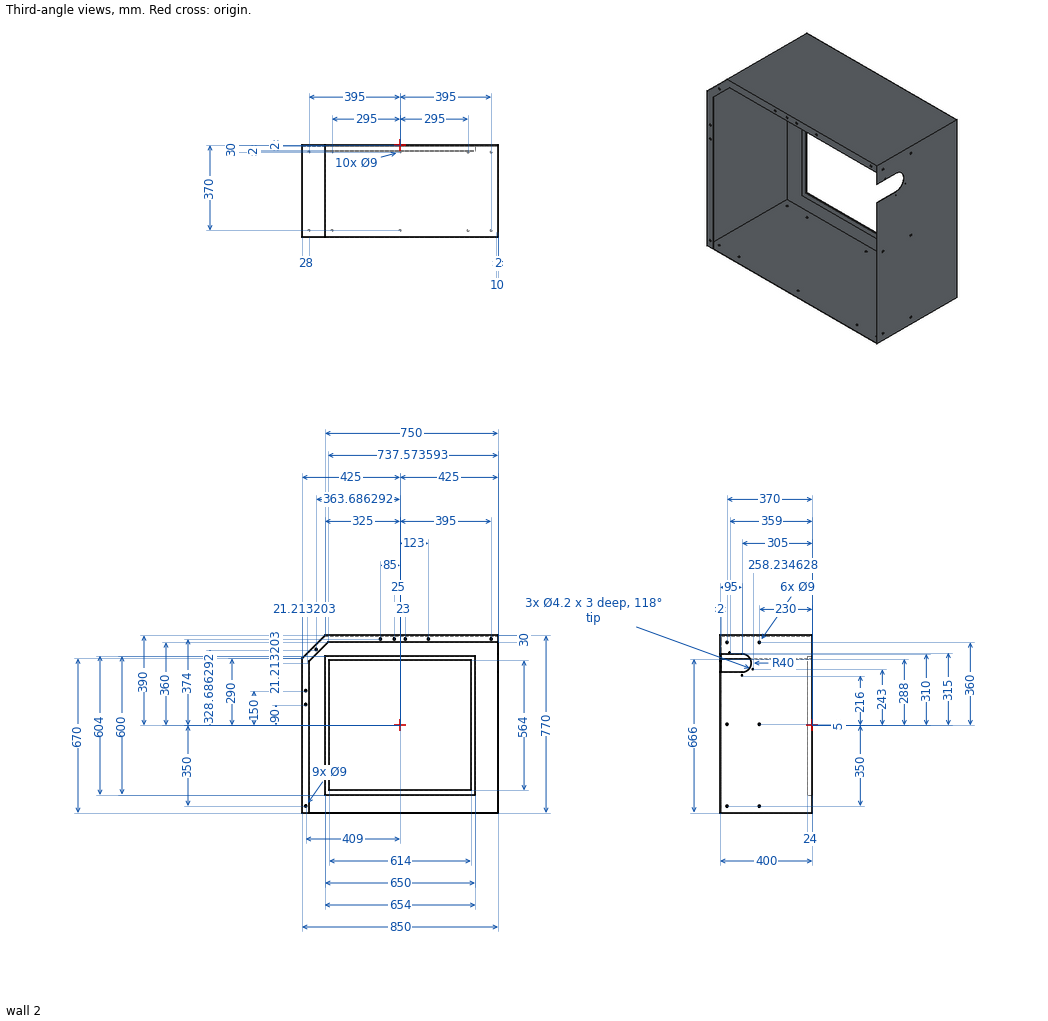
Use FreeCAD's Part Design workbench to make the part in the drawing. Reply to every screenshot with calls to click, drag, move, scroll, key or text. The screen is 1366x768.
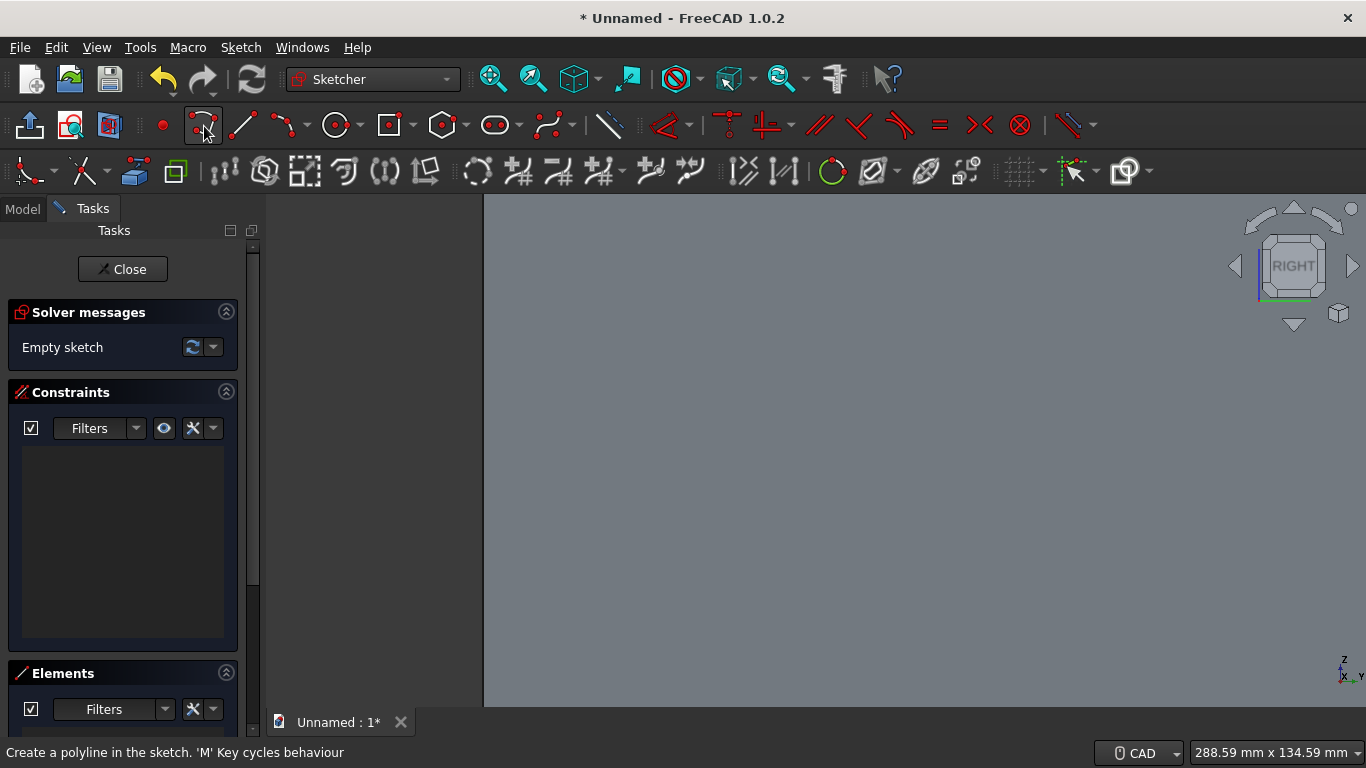
click(846, 293)
click(483, 293)
click(483, 598)
click(846, 598)
right_click(846, 598)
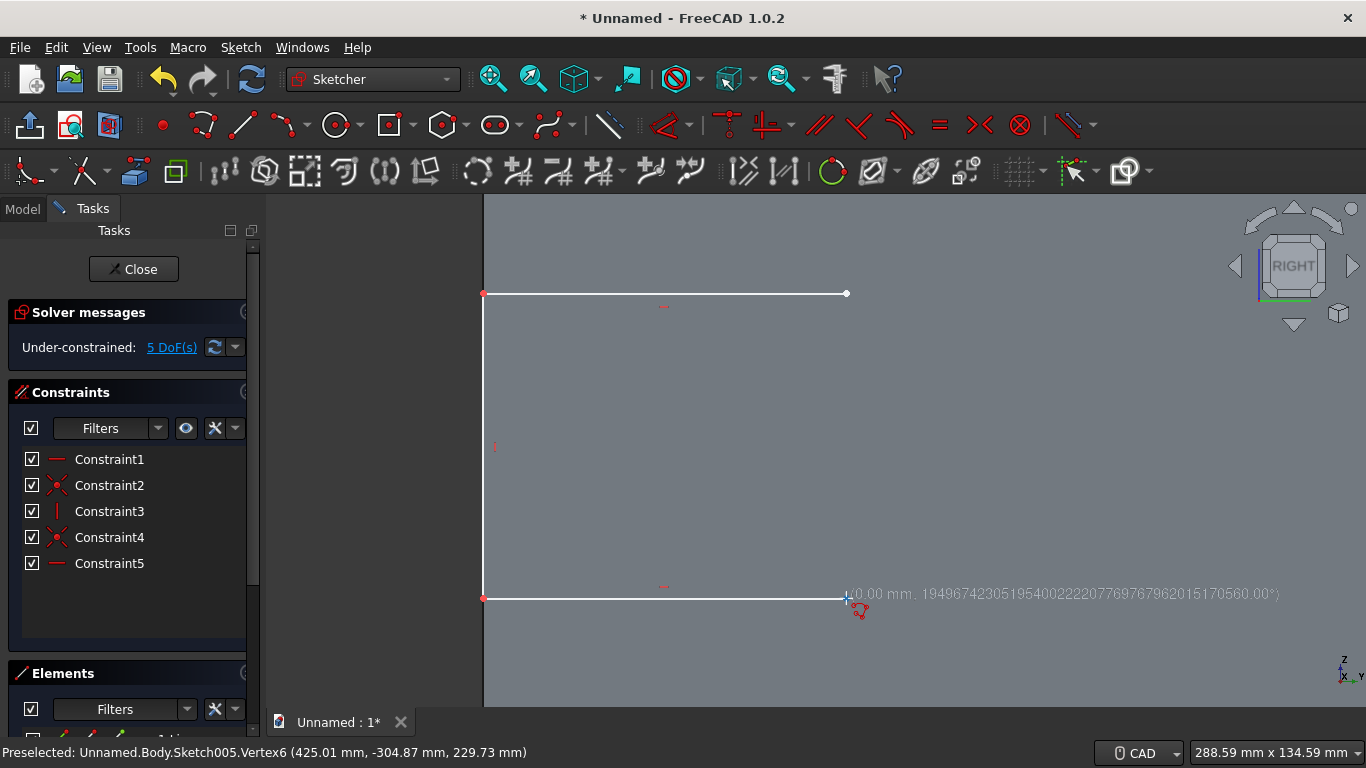
click(284, 126)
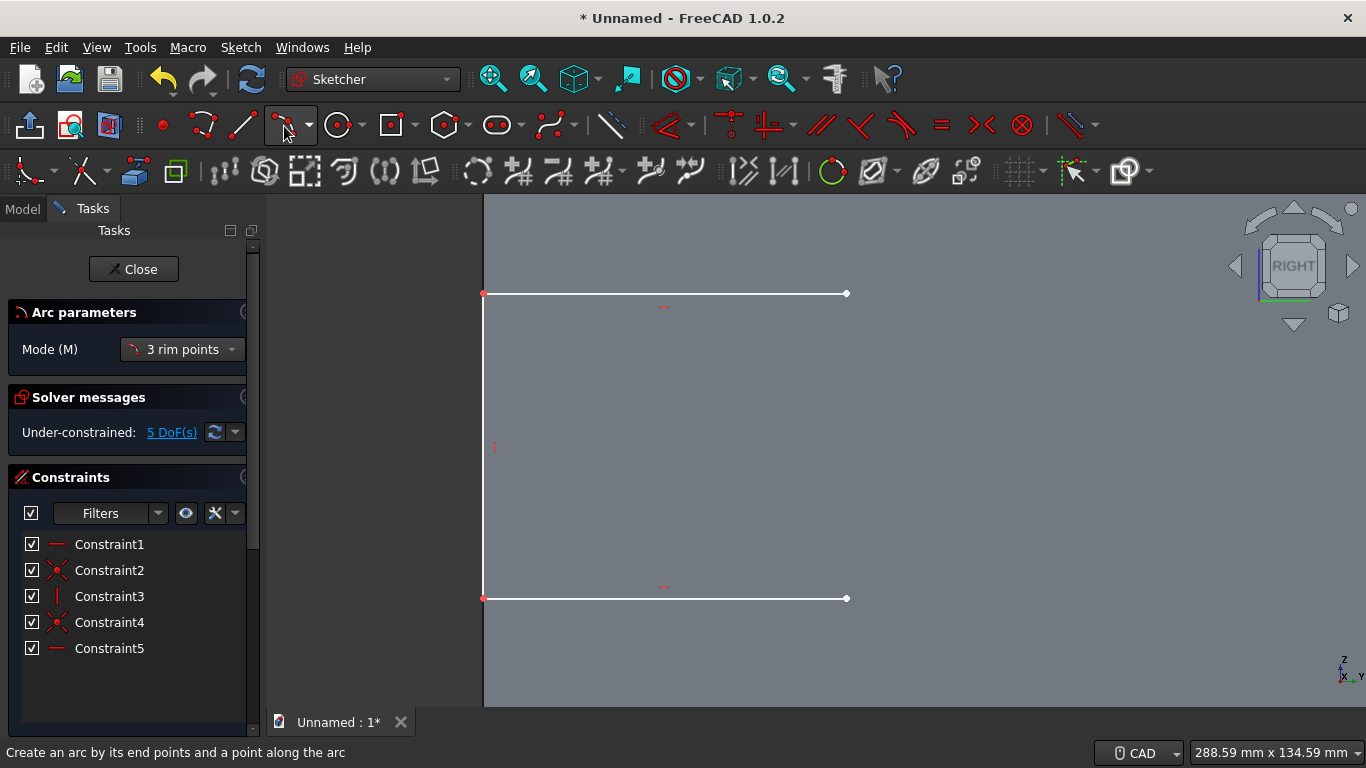
click(846, 599)
click(846, 294)
click(998, 446)
key(Escape)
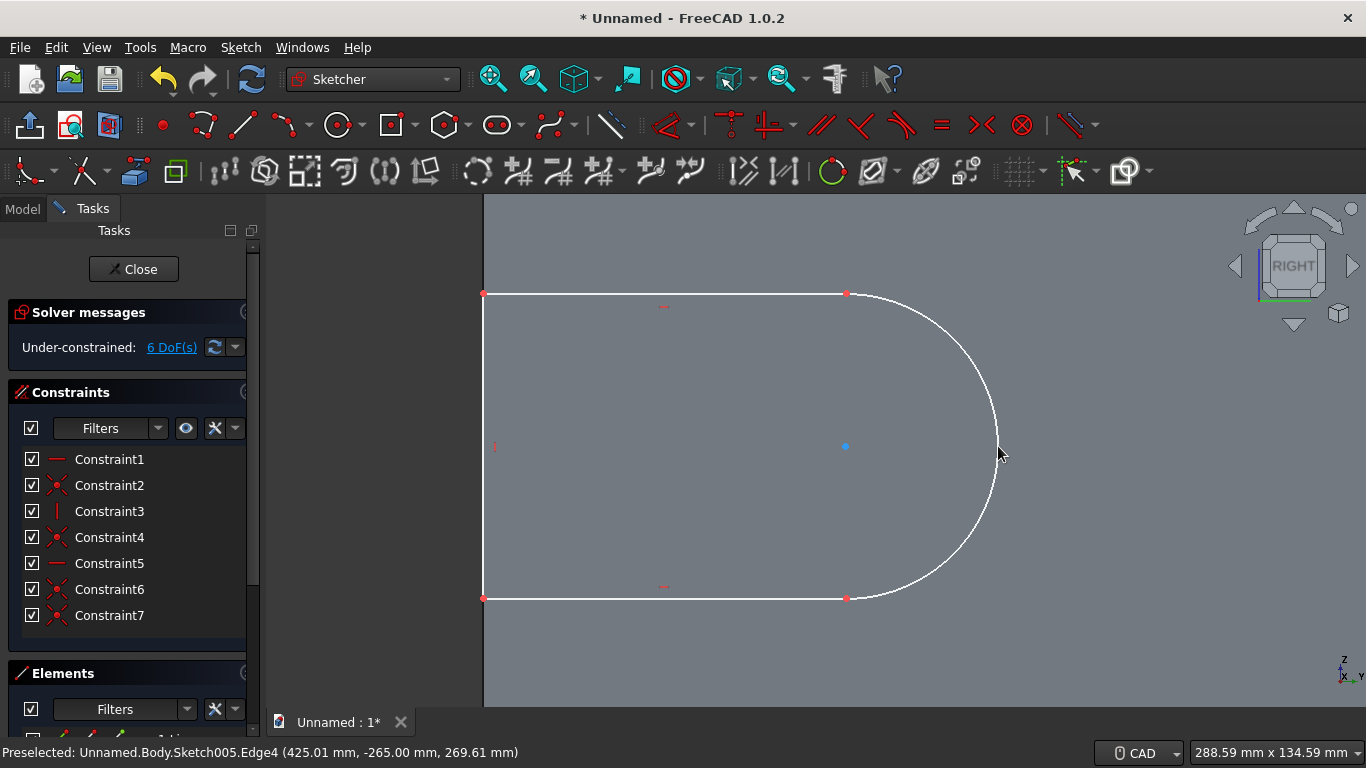
click(666, 126)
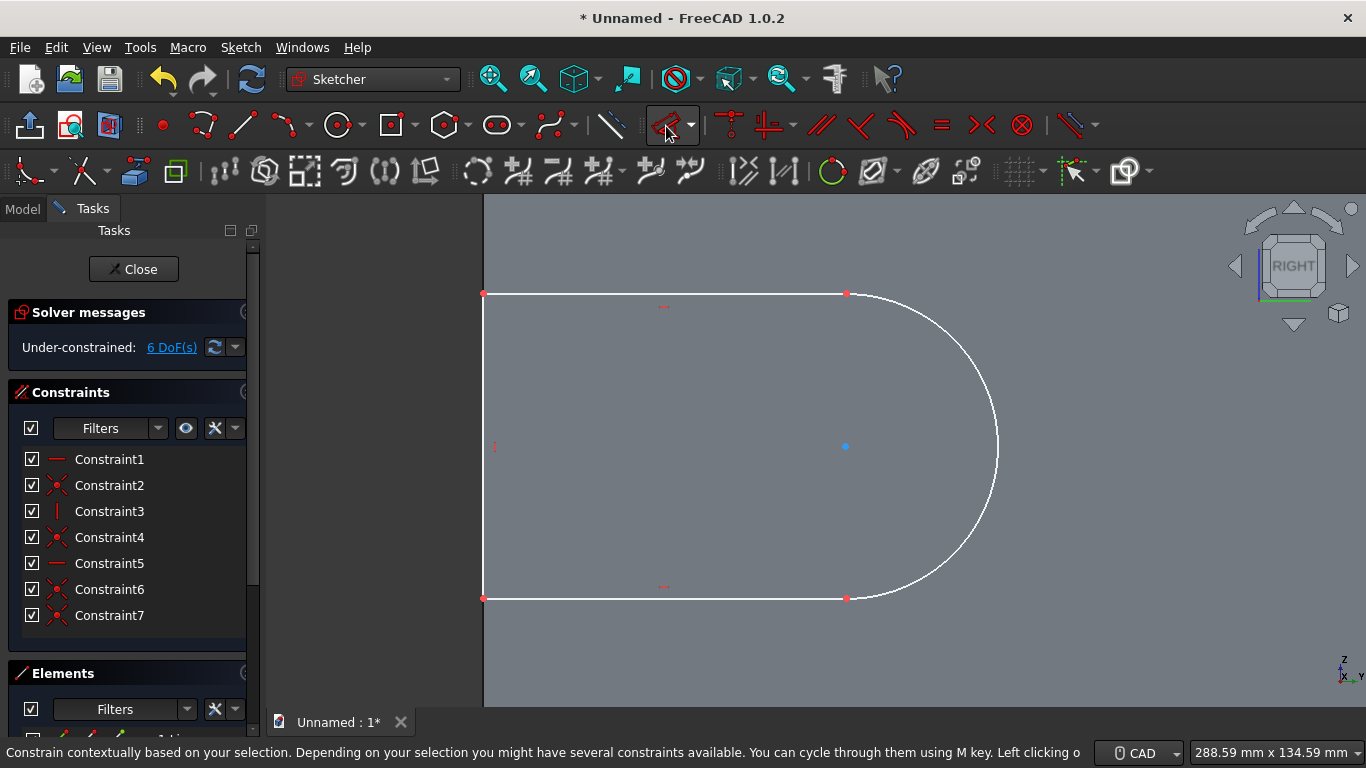
click(969, 536)
click(995, 555)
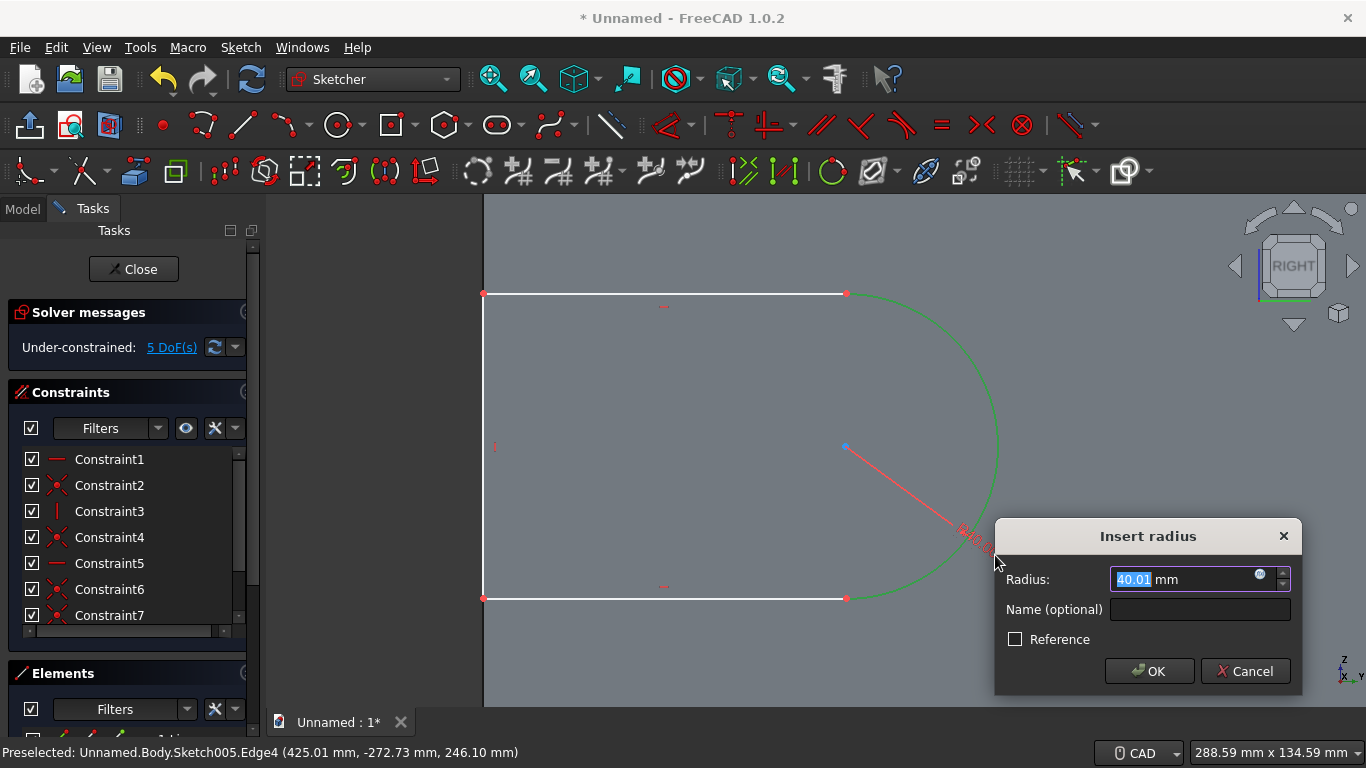
text(40)
key(Return)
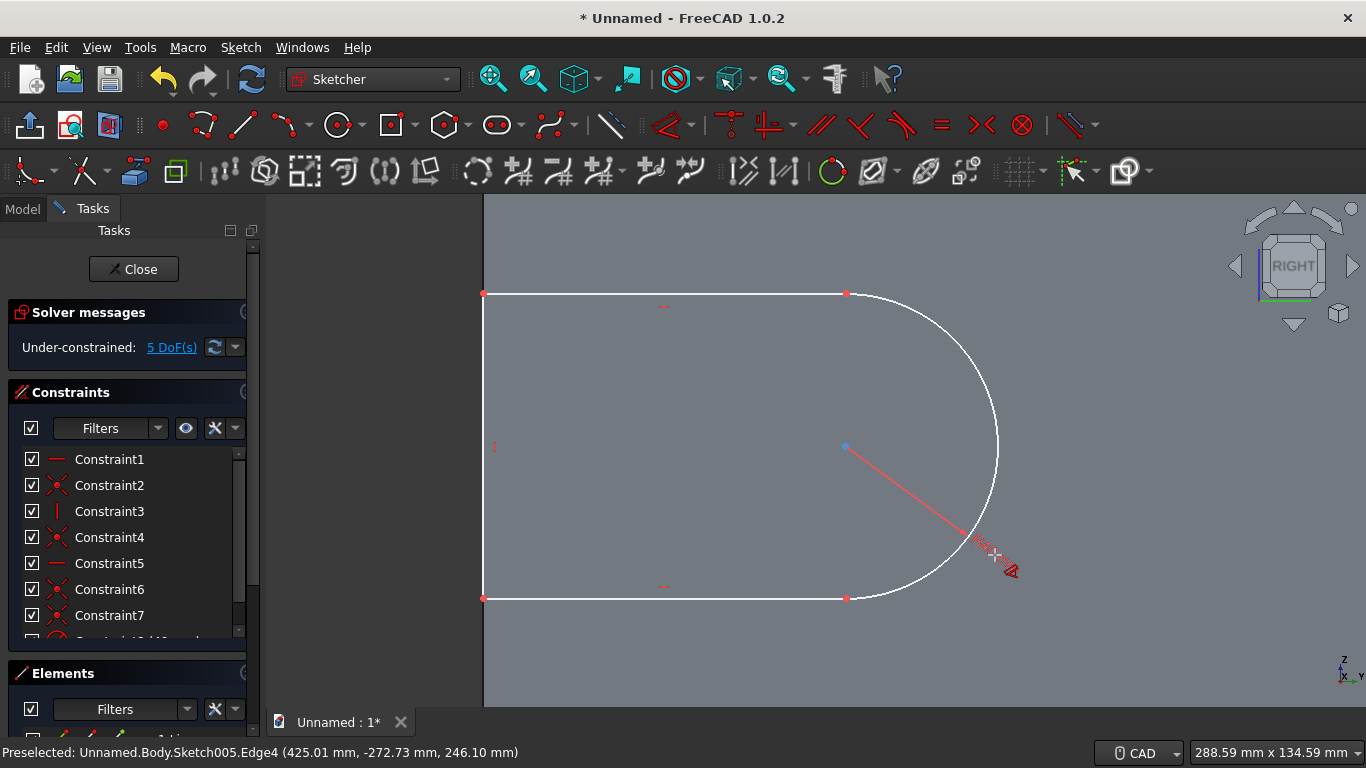
click(737, 294)
click(664, 260)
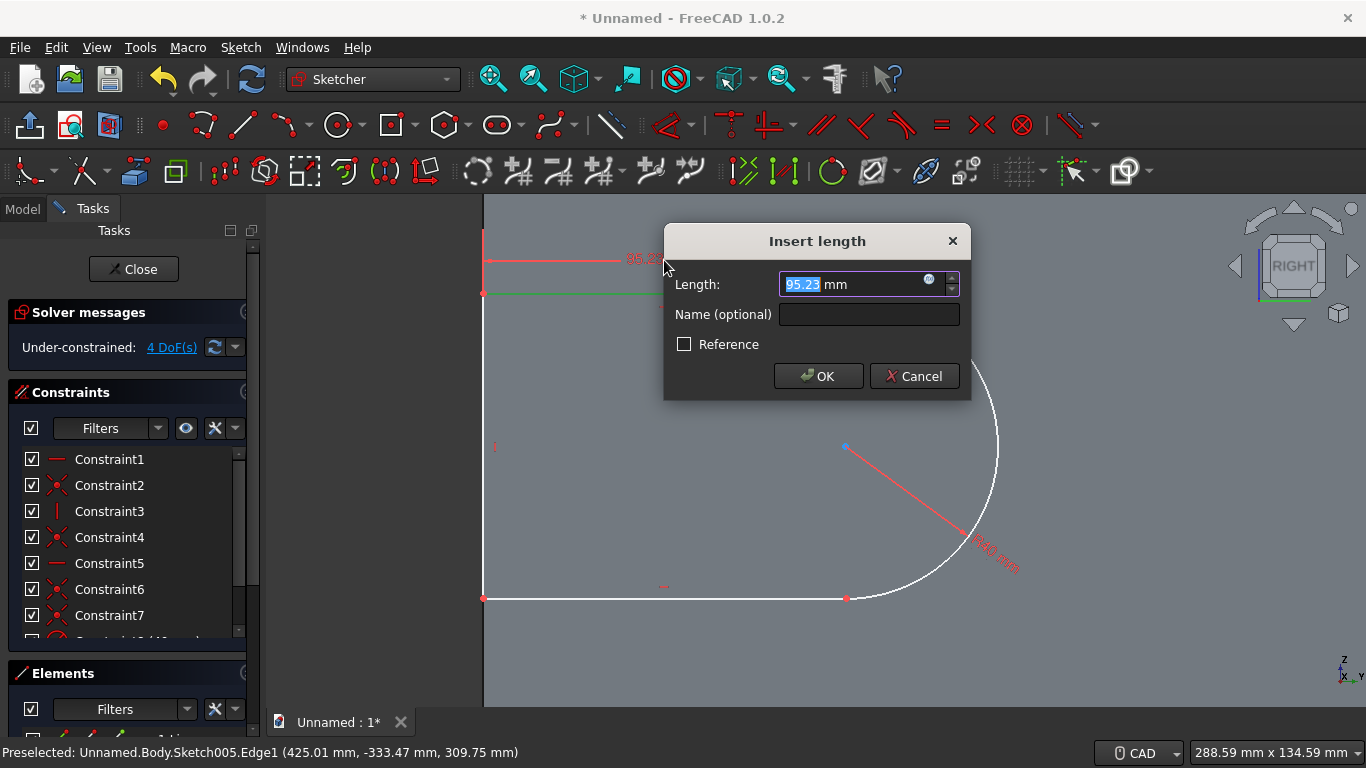
text(95)
key(Return)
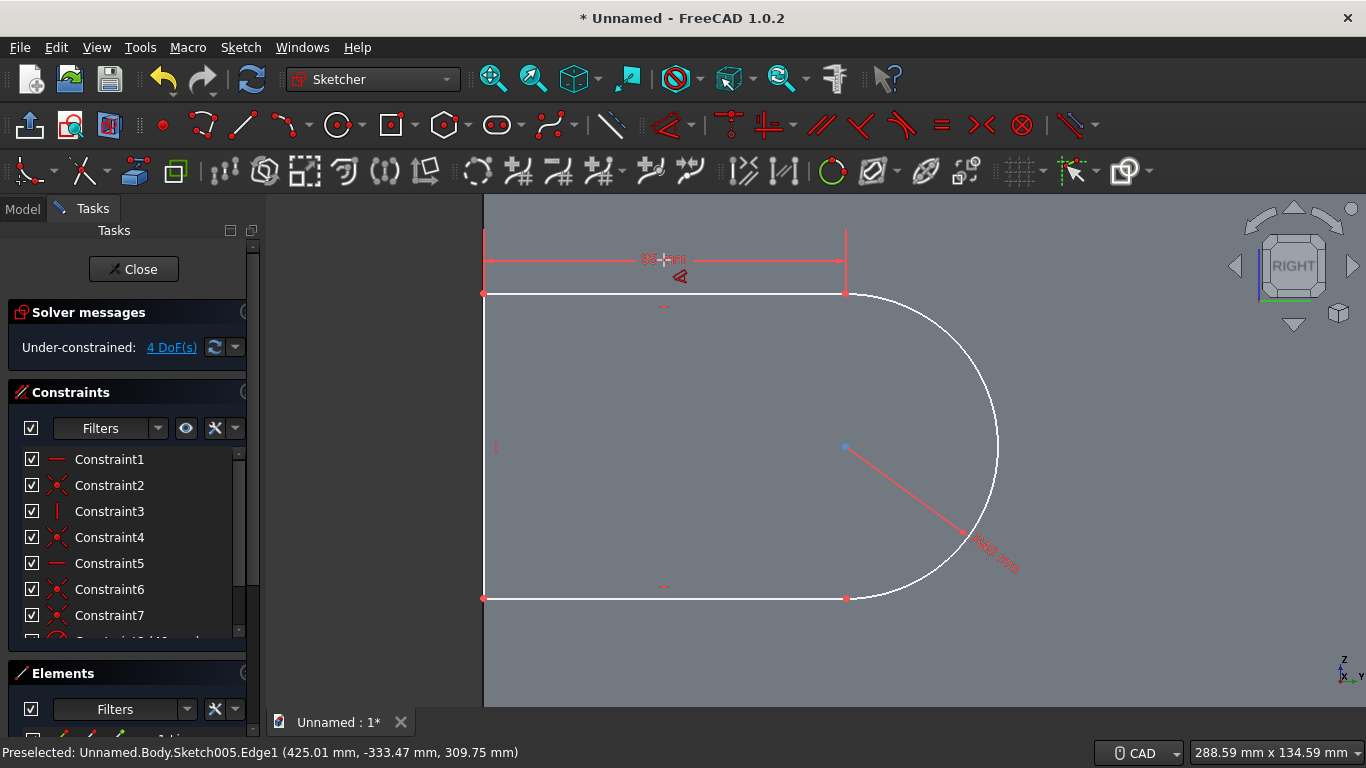
click(592, 599)
click(665, 633)